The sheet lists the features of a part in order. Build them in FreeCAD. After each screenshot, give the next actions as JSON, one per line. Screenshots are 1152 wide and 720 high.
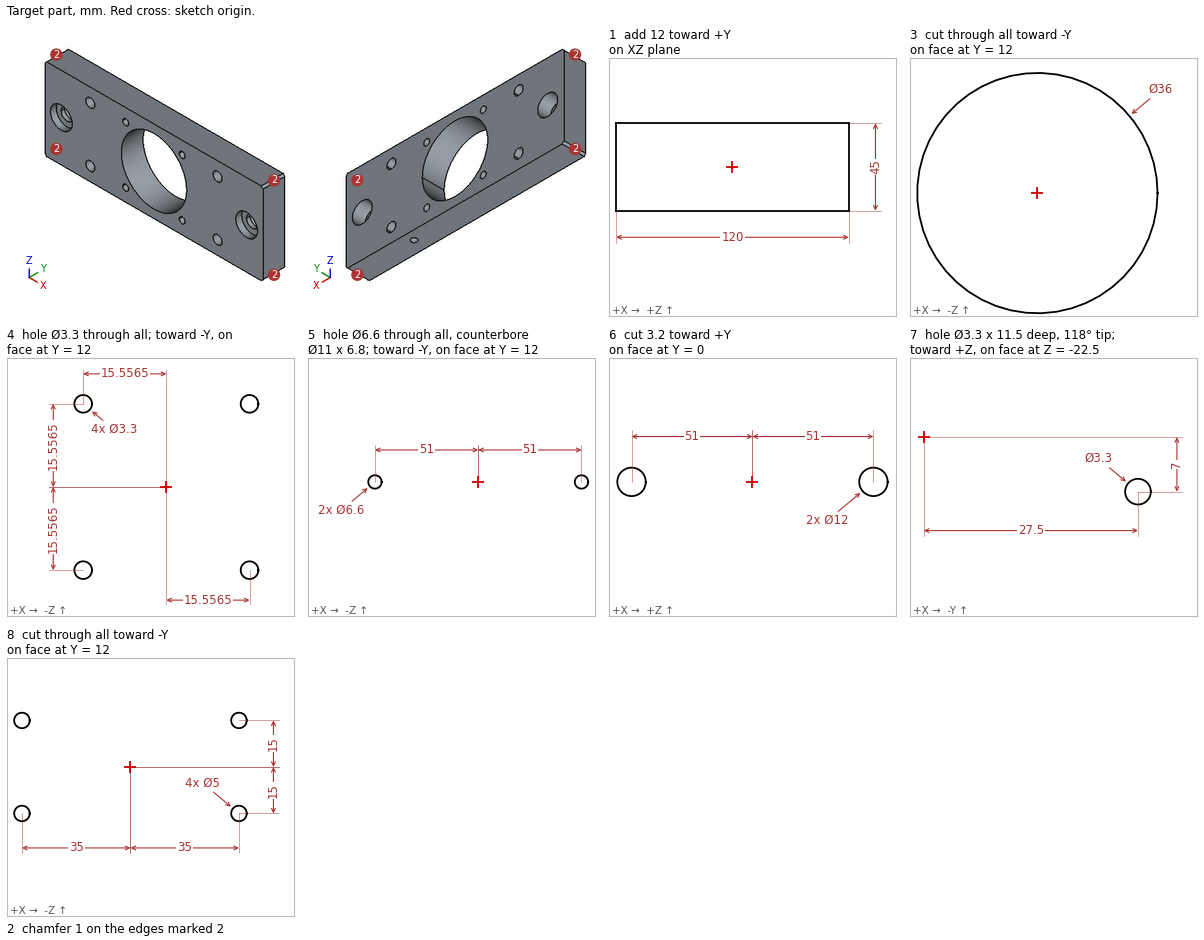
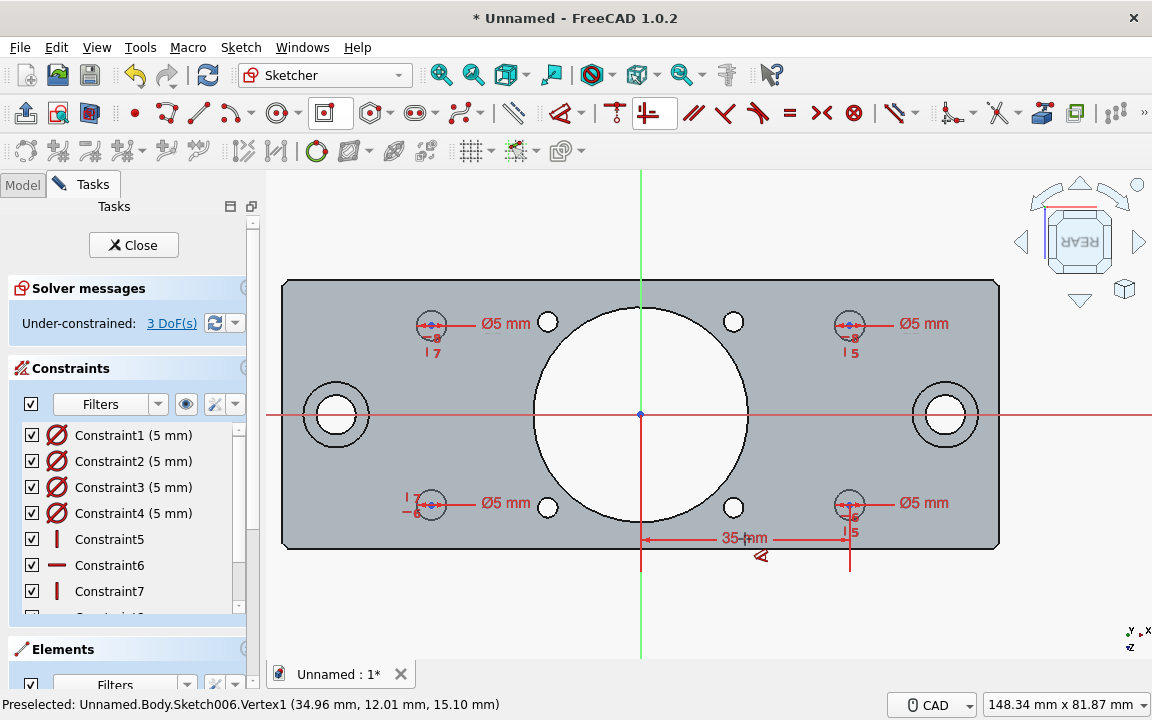
{"action": "left_click", "coordinate": [850, 505]}
{"action": "left_click", "coordinate": [884, 460]}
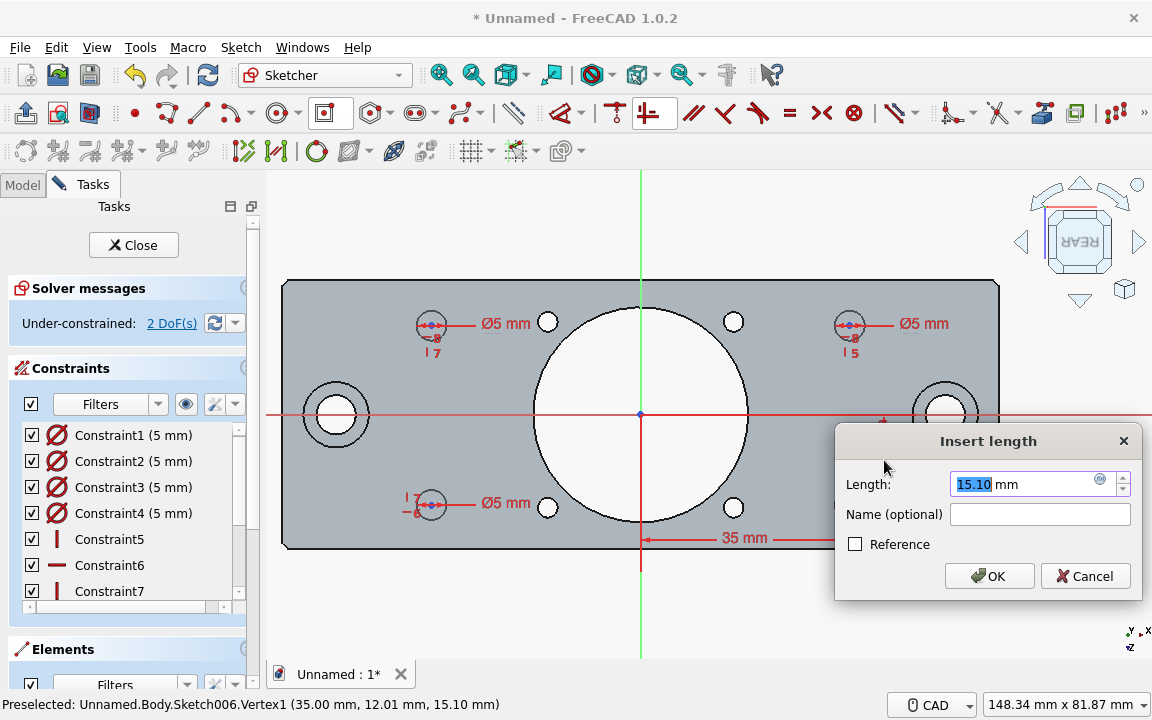
{"action": "type", "text": "15"}
{"action": "key", "text": "Return"}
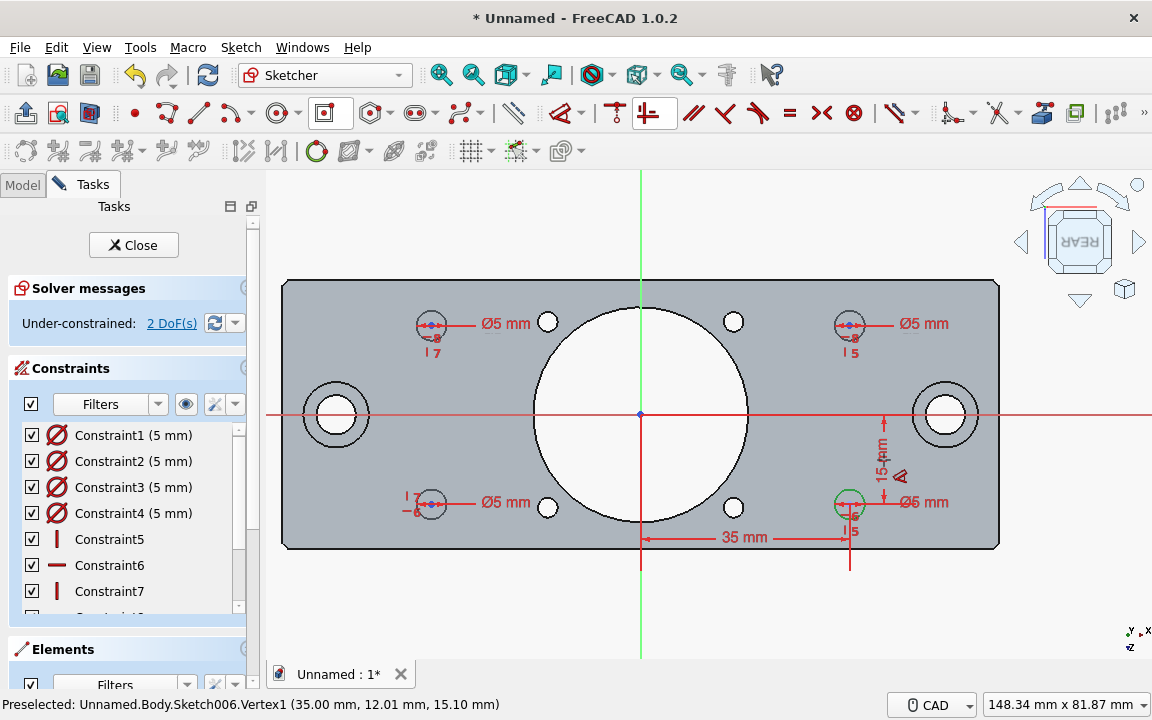
{"action": "left_click", "coordinate": [850, 326]}
{"action": "left_click", "coordinate": [884, 370]}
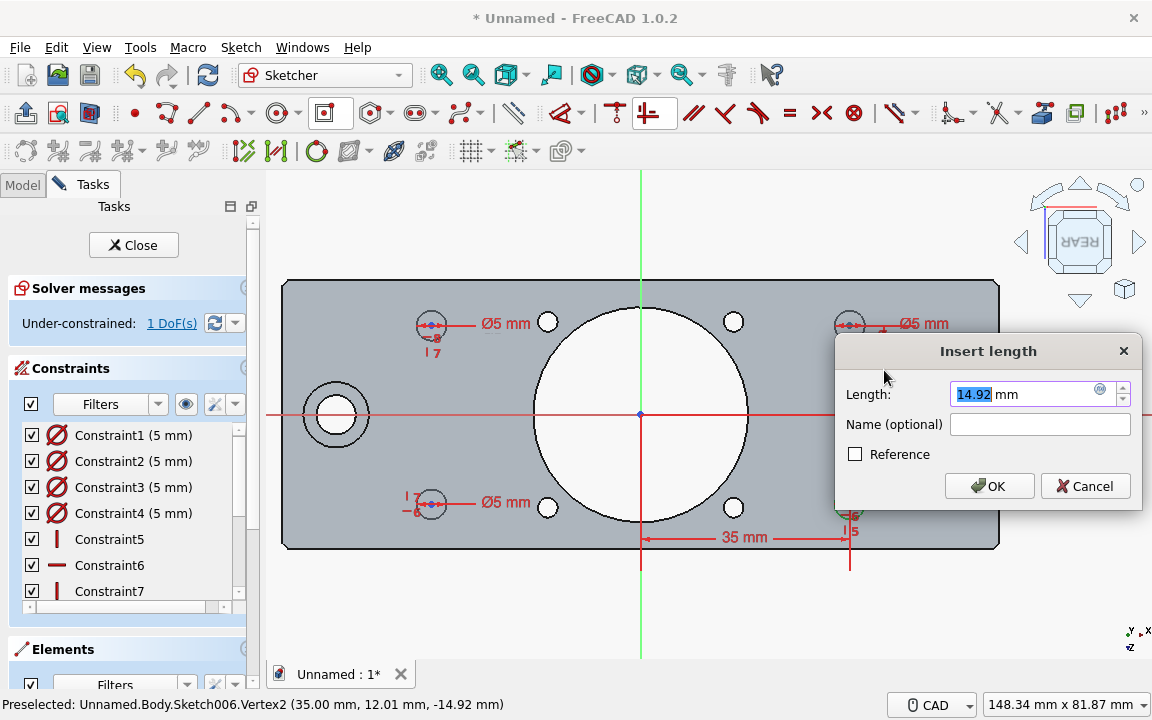
{"action": "type", "text": "15"}
{"action": "key", "text": "Return"}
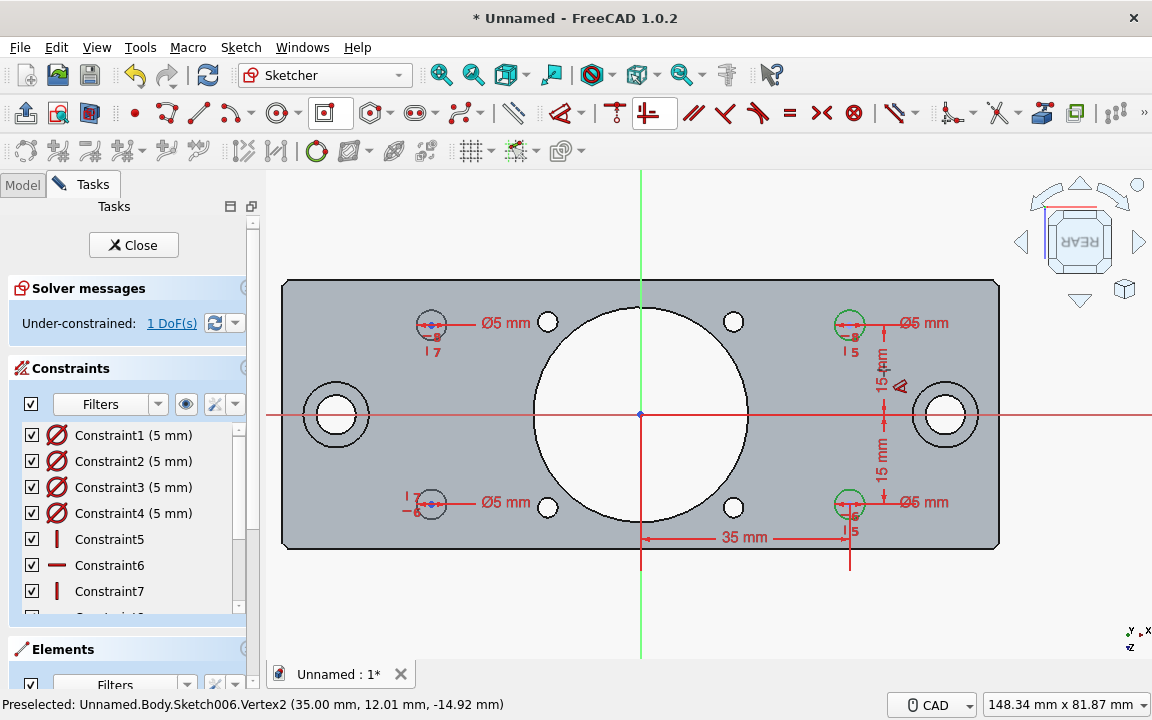
{"action": "left_click", "coordinate": [432, 504]}
{"action": "left_click", "coordinate": [536, 538]}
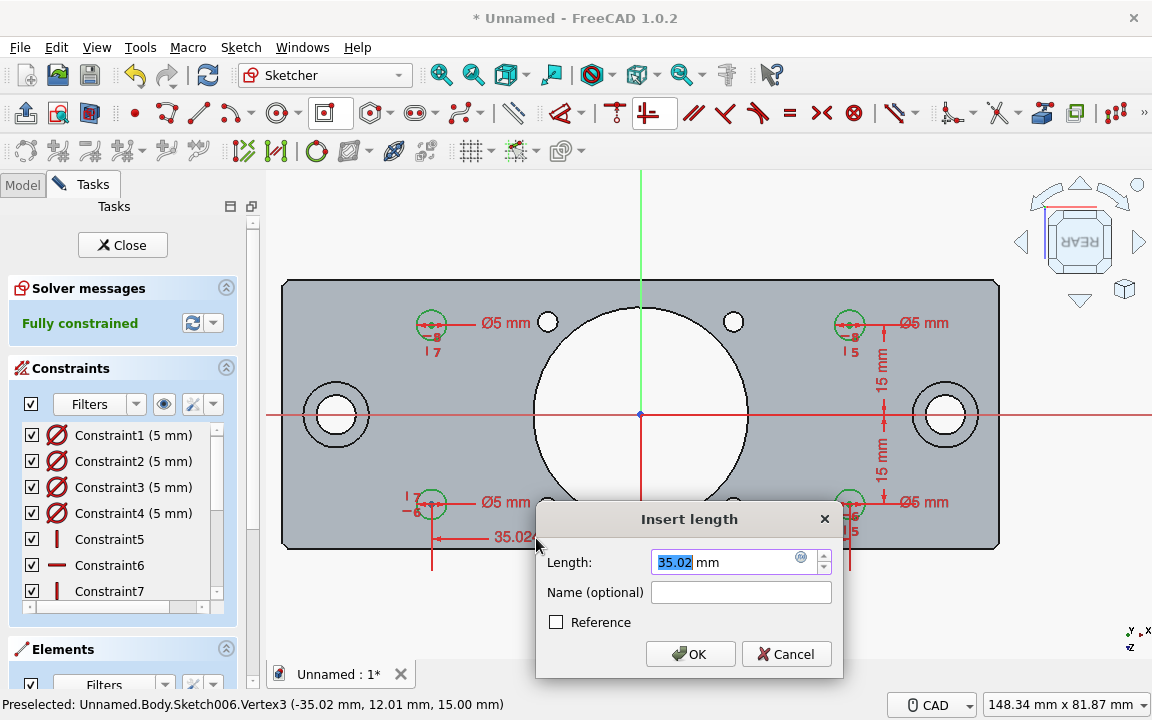
{"action": "type", "text": "35"}
{"action": "key", "text": "Return"}
{"action": "key", "text": "Escape"}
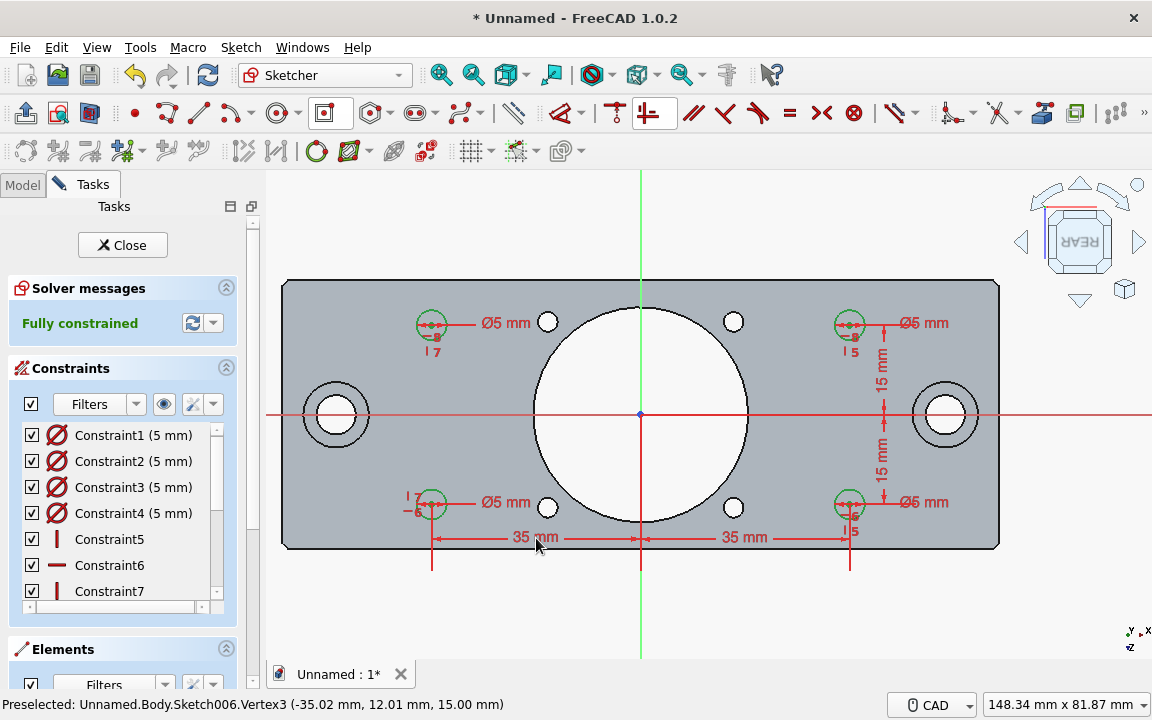
{"action": "left_click", "coordinate": [123, 245]}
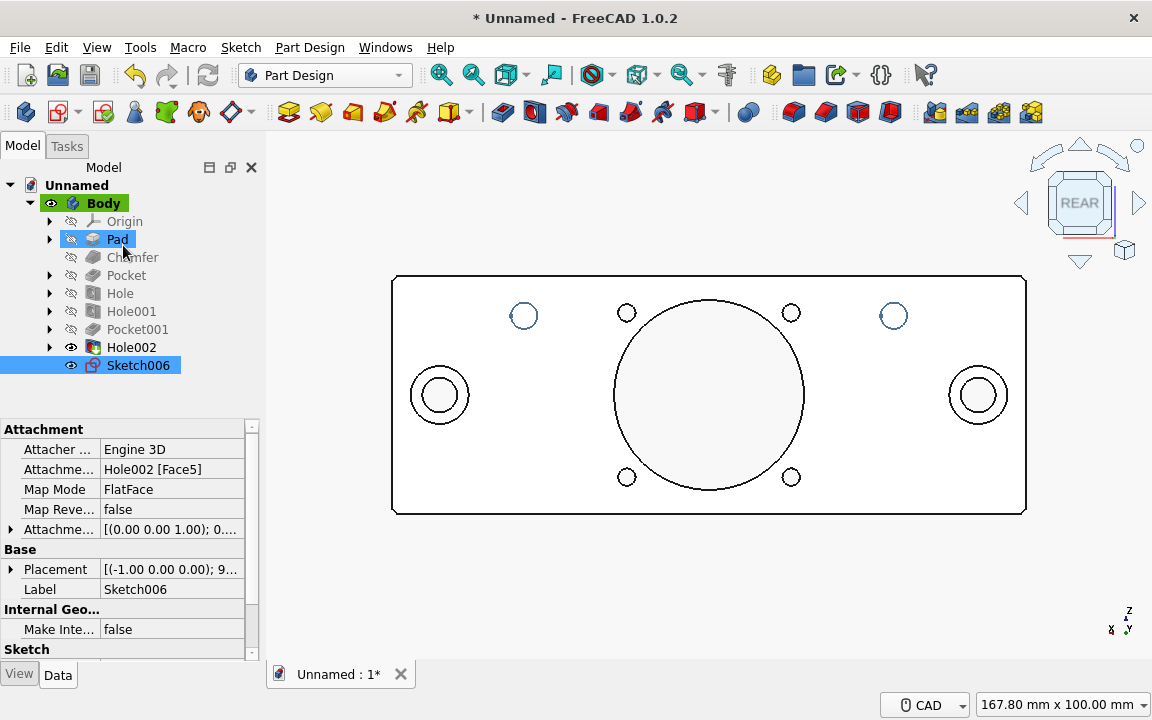
{"action": "left_click", "coordinate": [504, 112]}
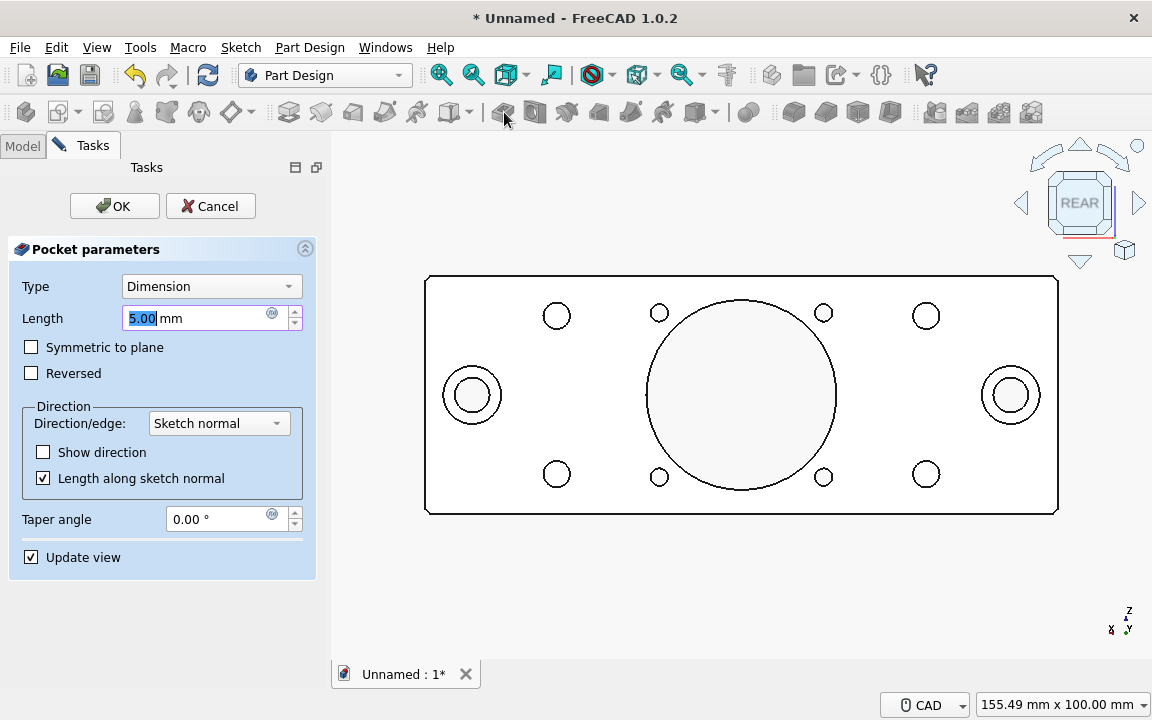
{"action": "left_click", "coordinate": [212, 286]}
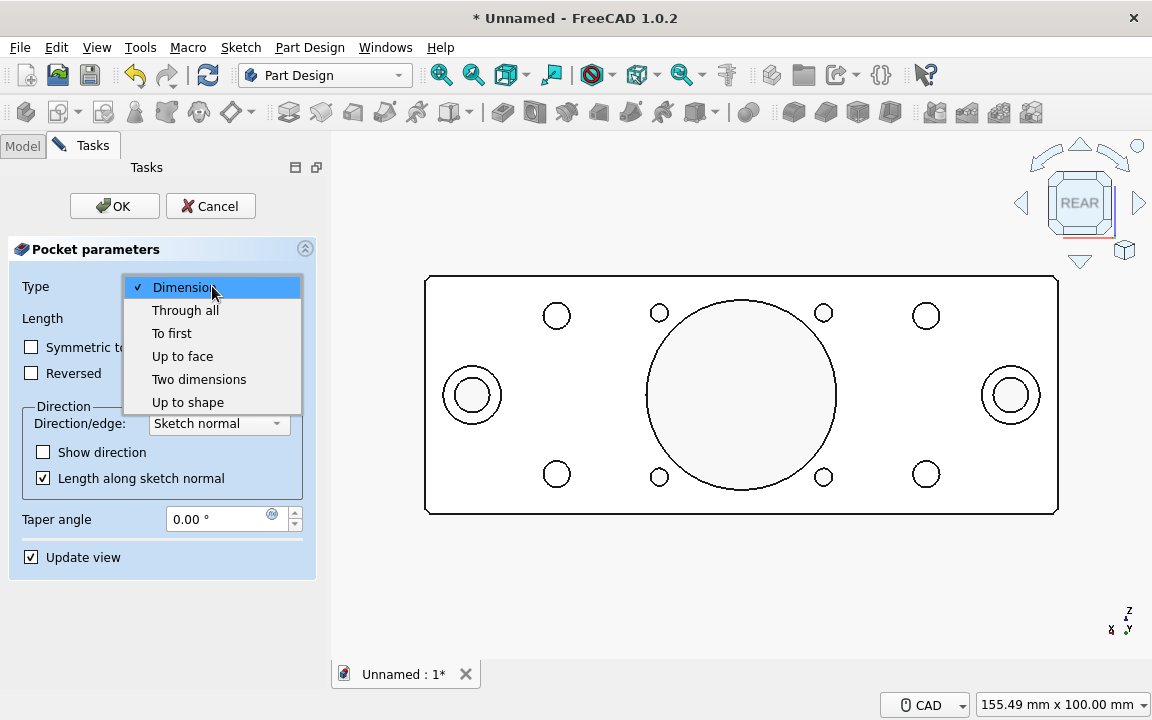
{"action": "left_click", "coordinate": [212, 310]}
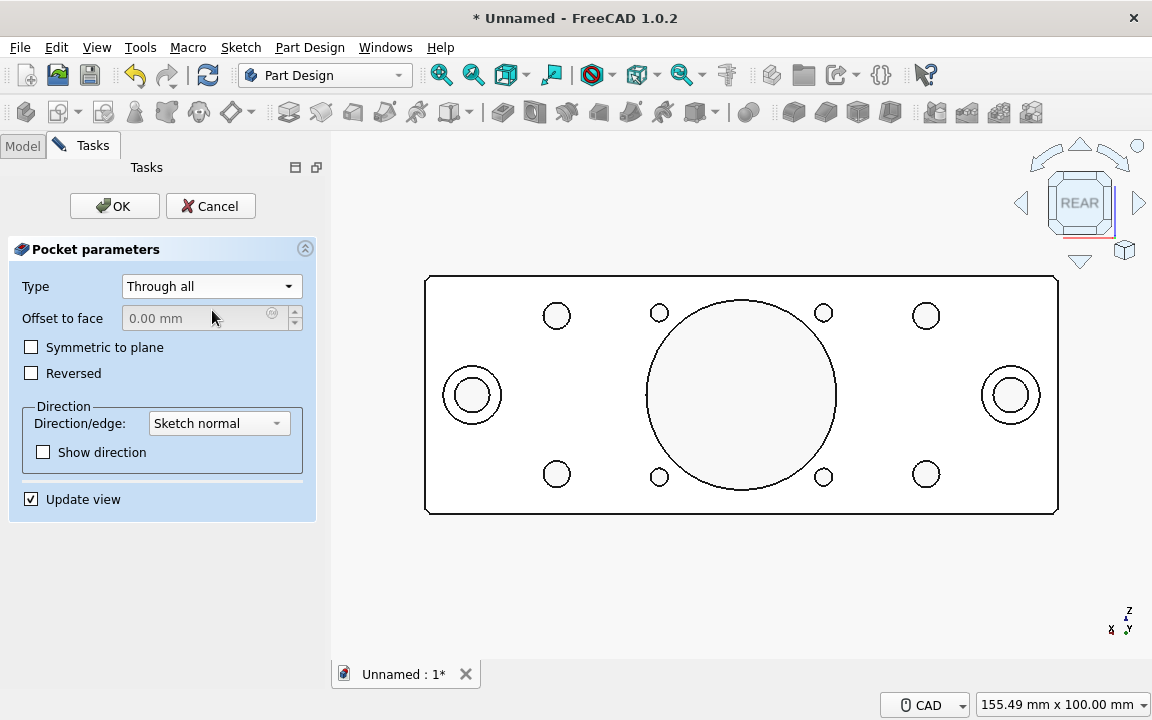
{"action": "left_click", "coordinate": [115, 206]}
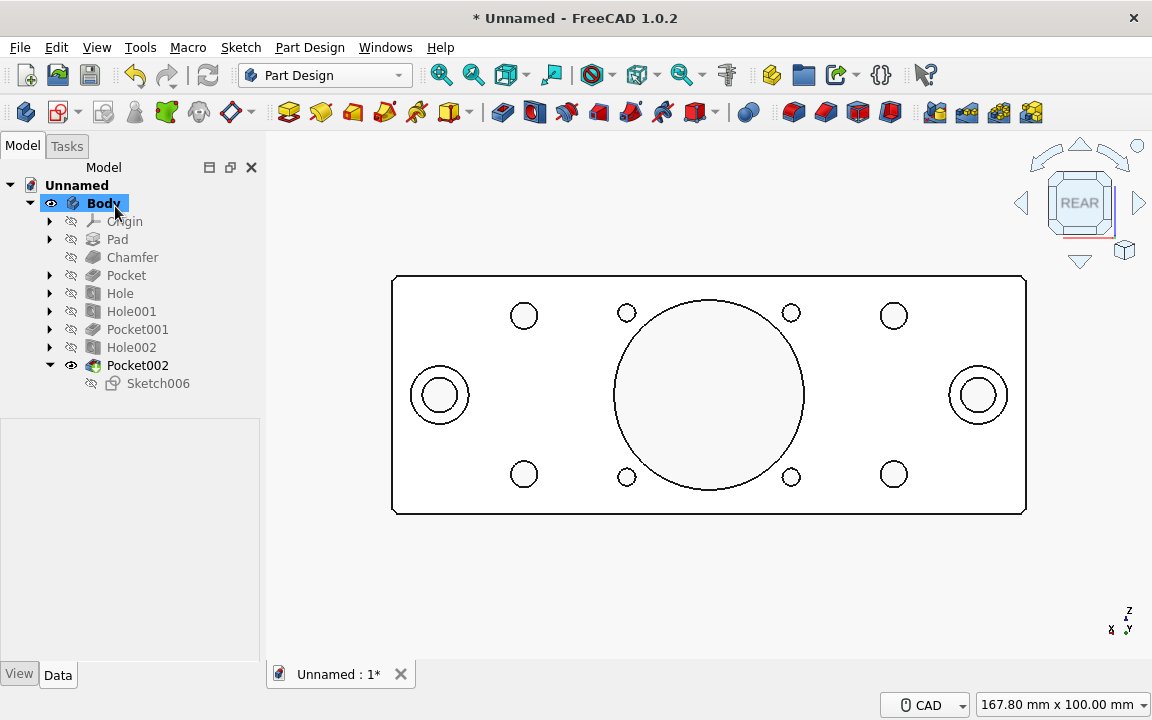
{"action": "key", "text": "0"}